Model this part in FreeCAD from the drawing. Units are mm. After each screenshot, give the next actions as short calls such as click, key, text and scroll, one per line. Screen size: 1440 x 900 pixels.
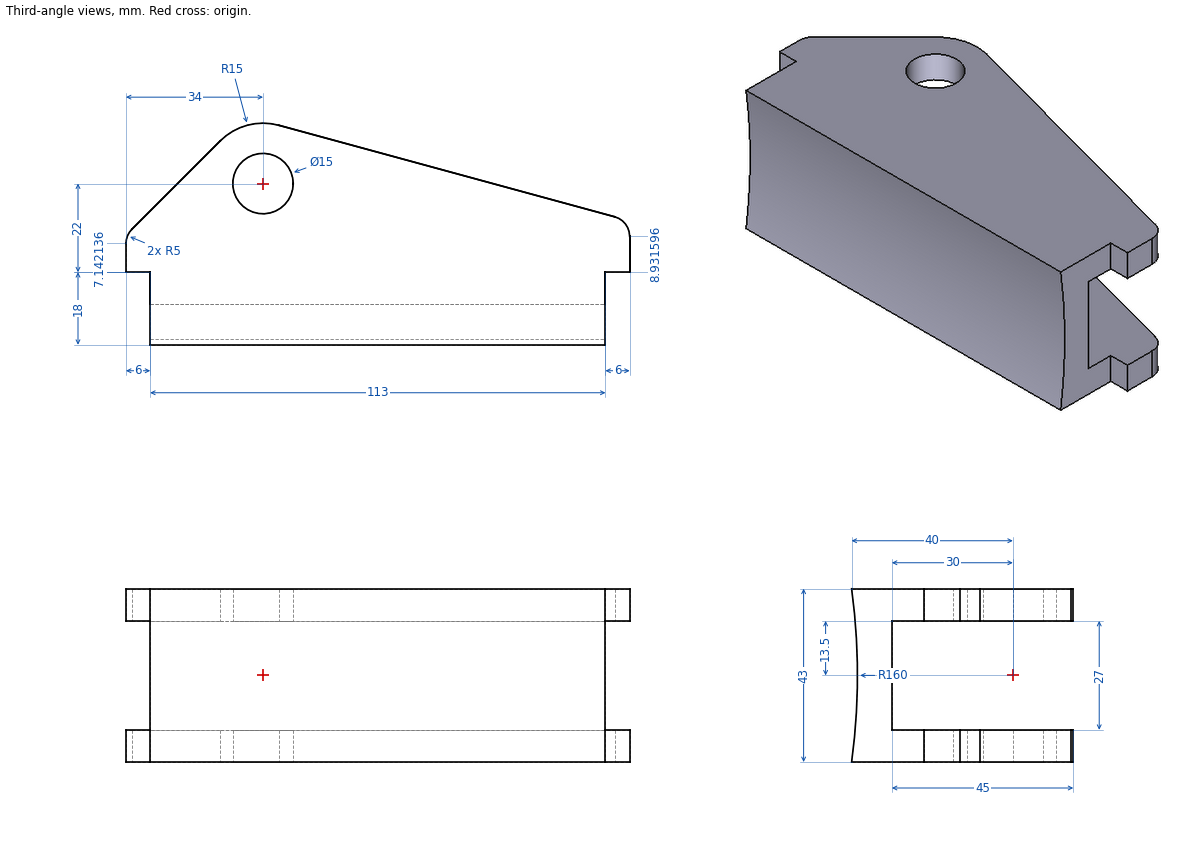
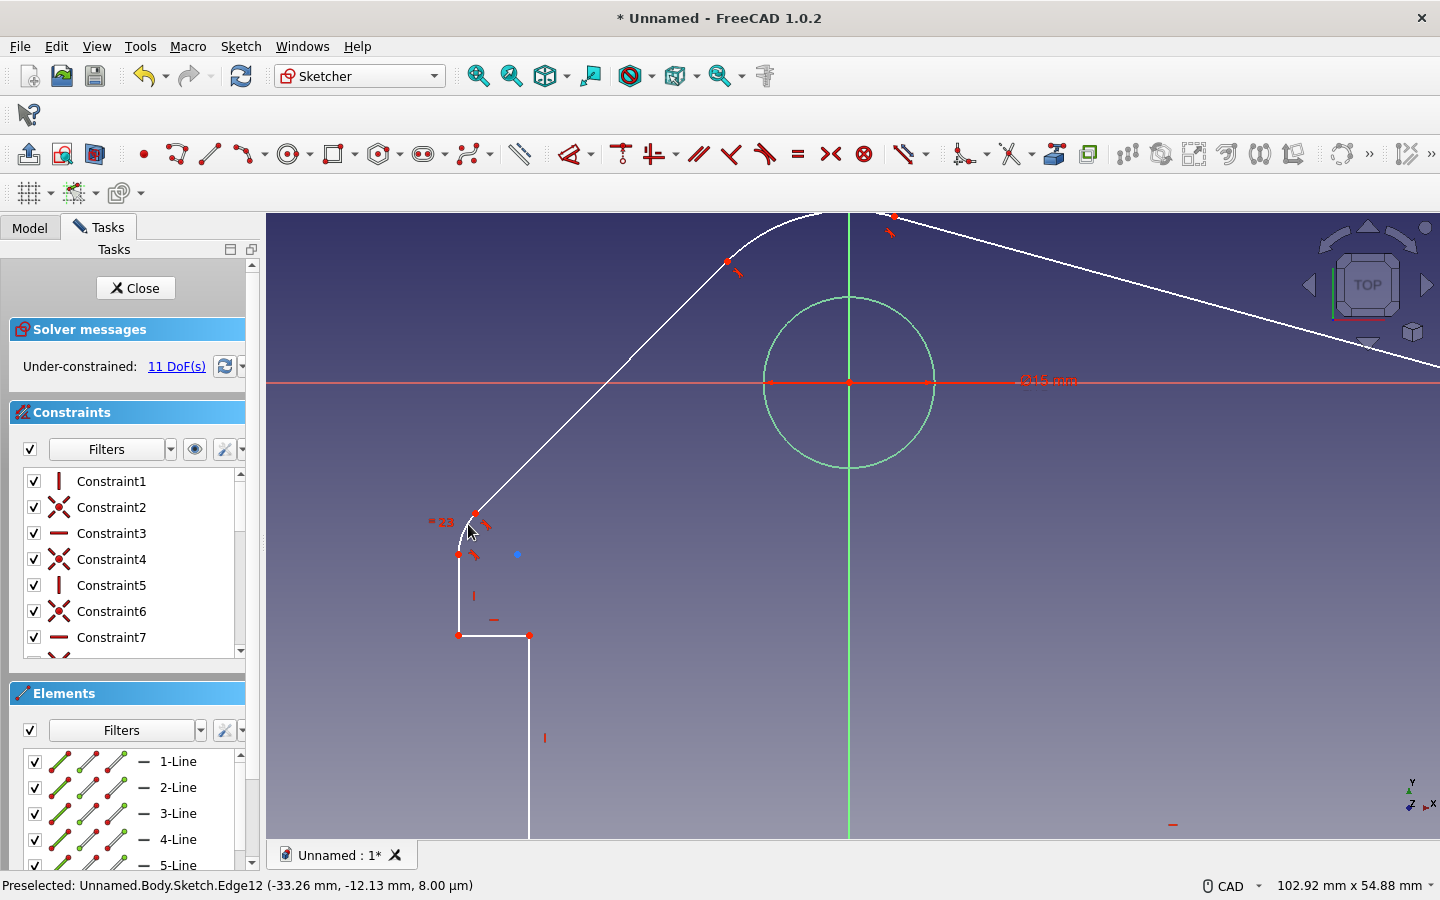
click(568, 154)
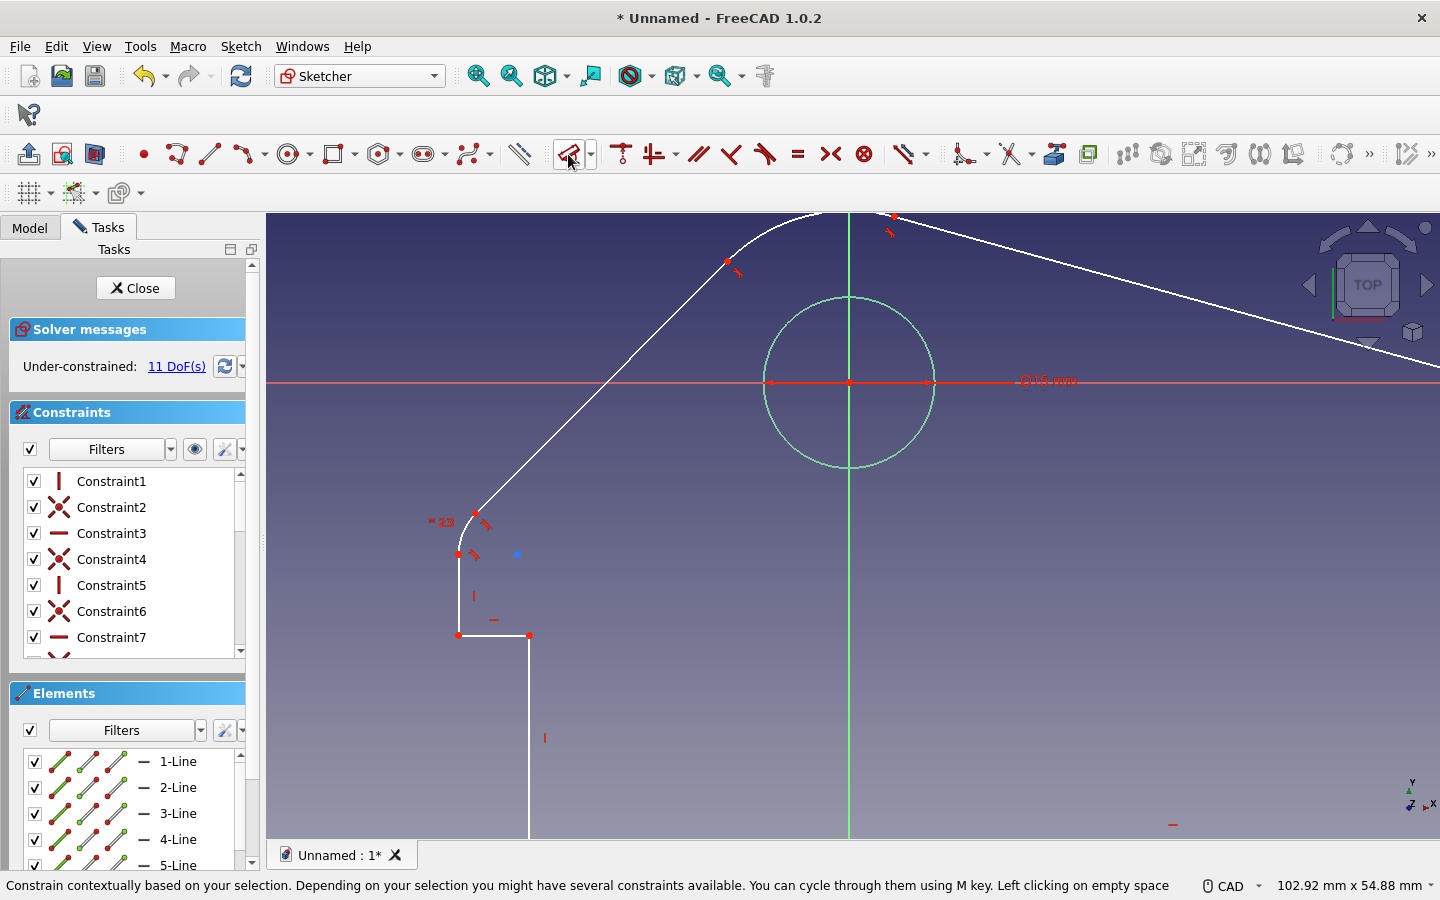
scroll(467, 524, down, 4)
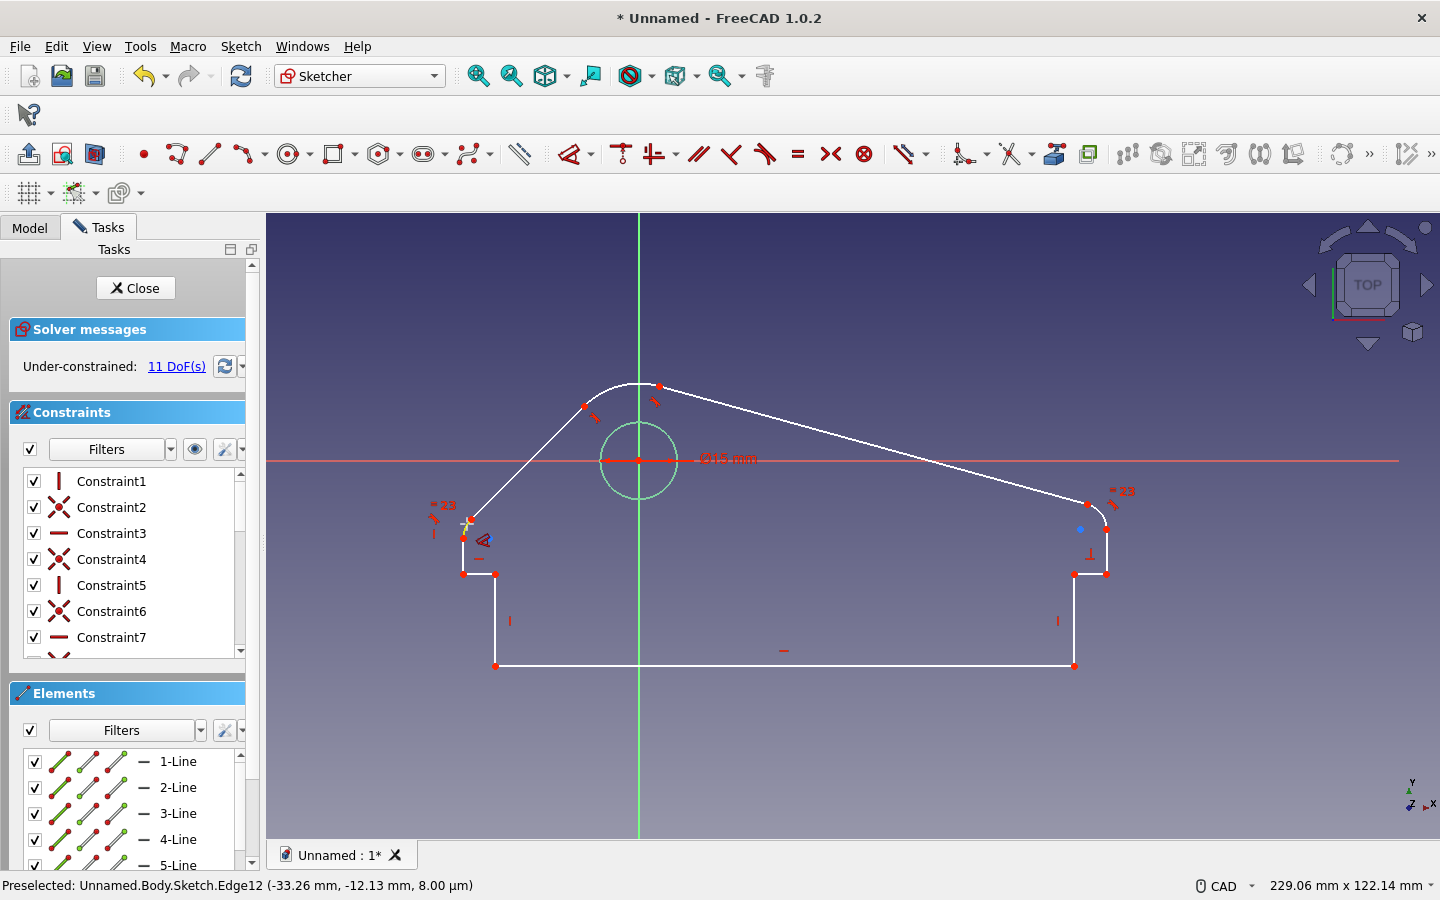
scroll(1105, 520, up, 3)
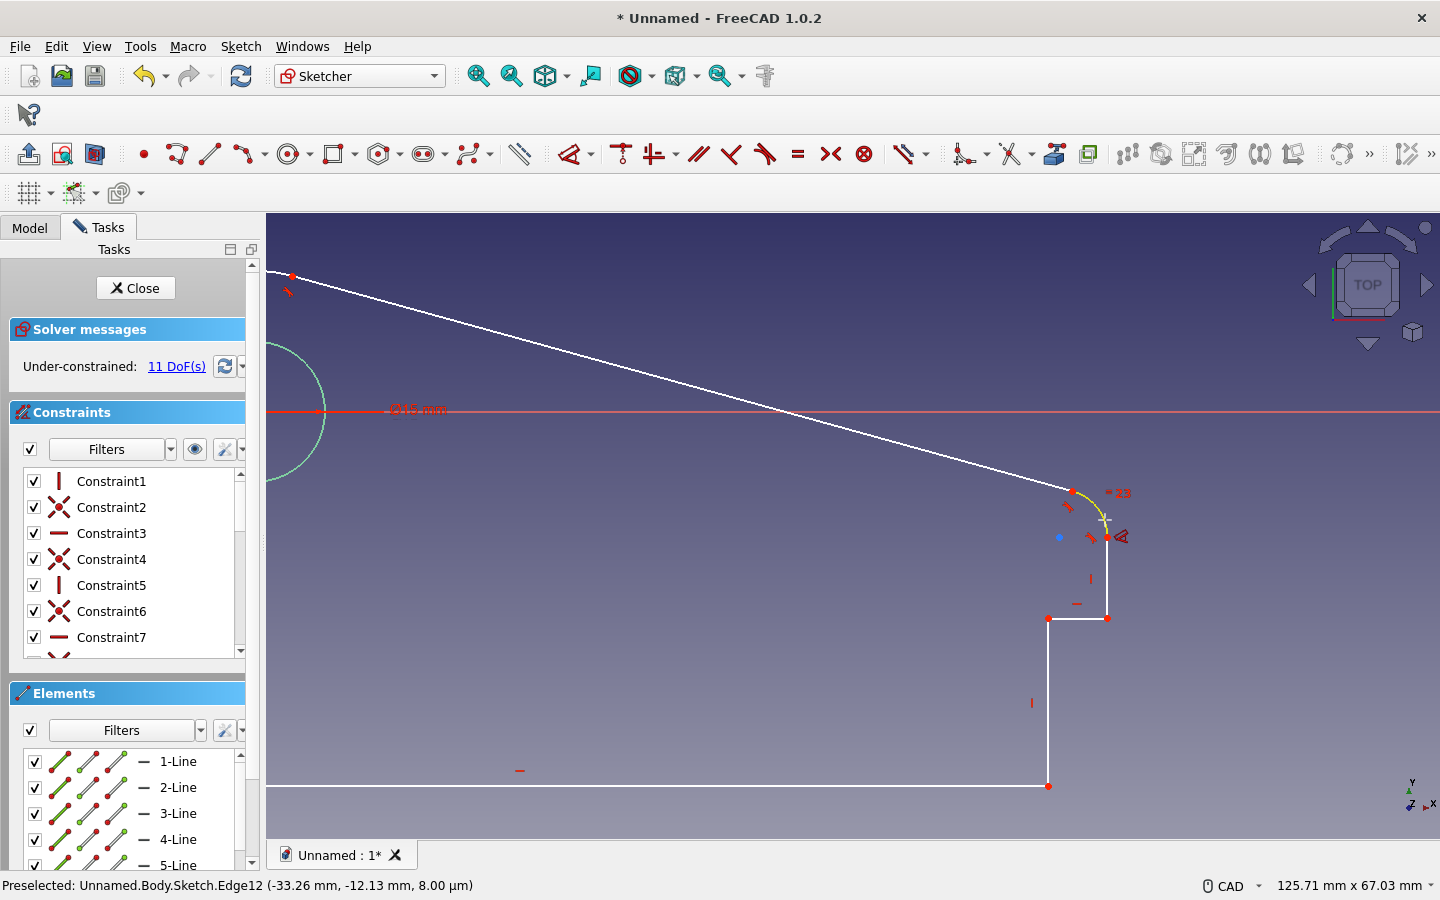
click(1104, 519)
click(1134, 507)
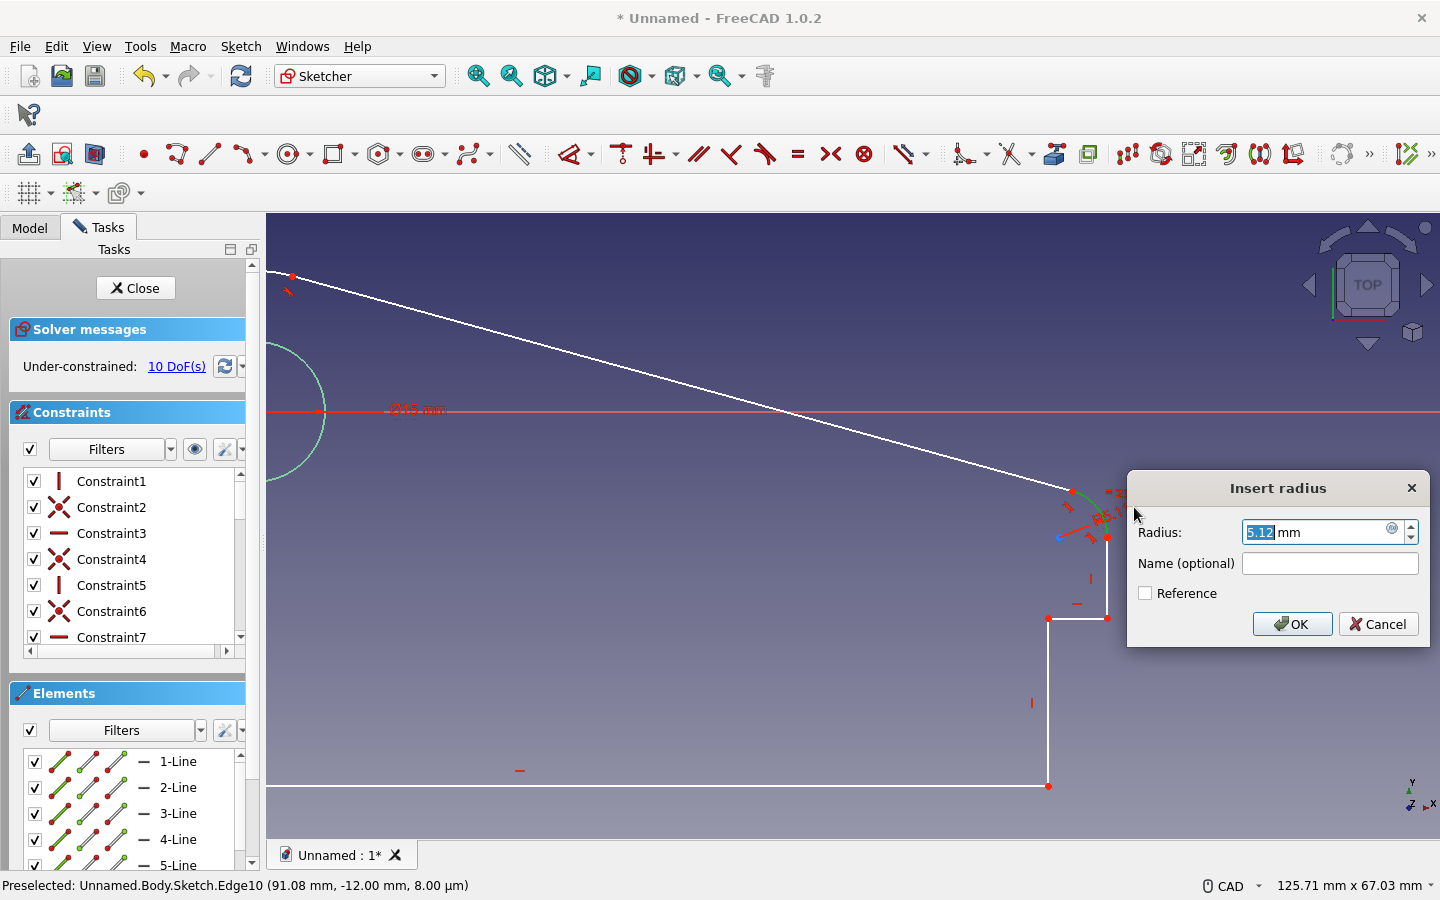
text(5)
key(Return)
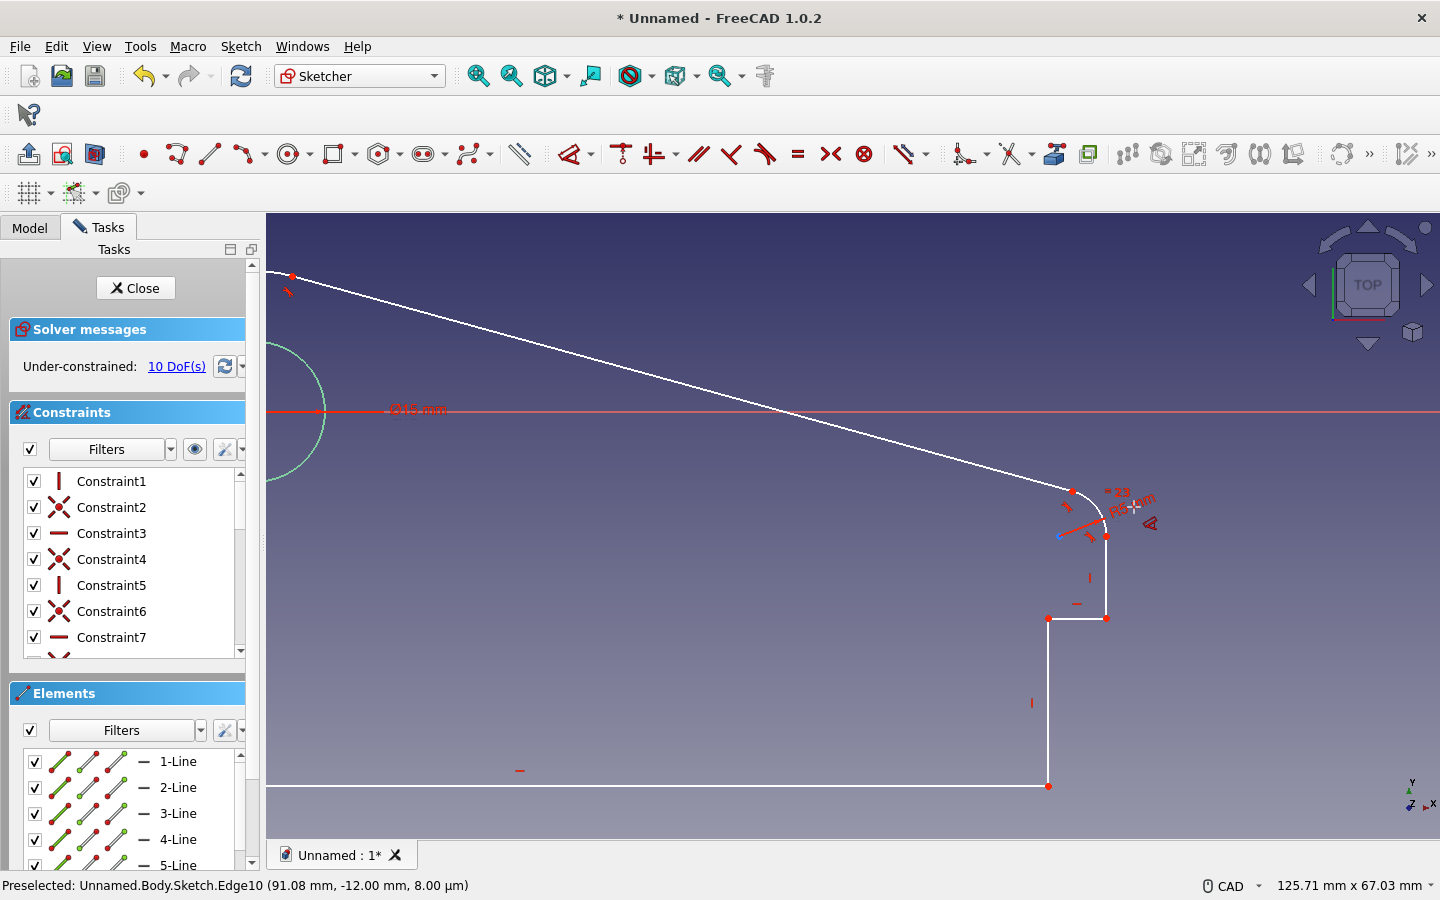
scroll(1105, 520, down, 3)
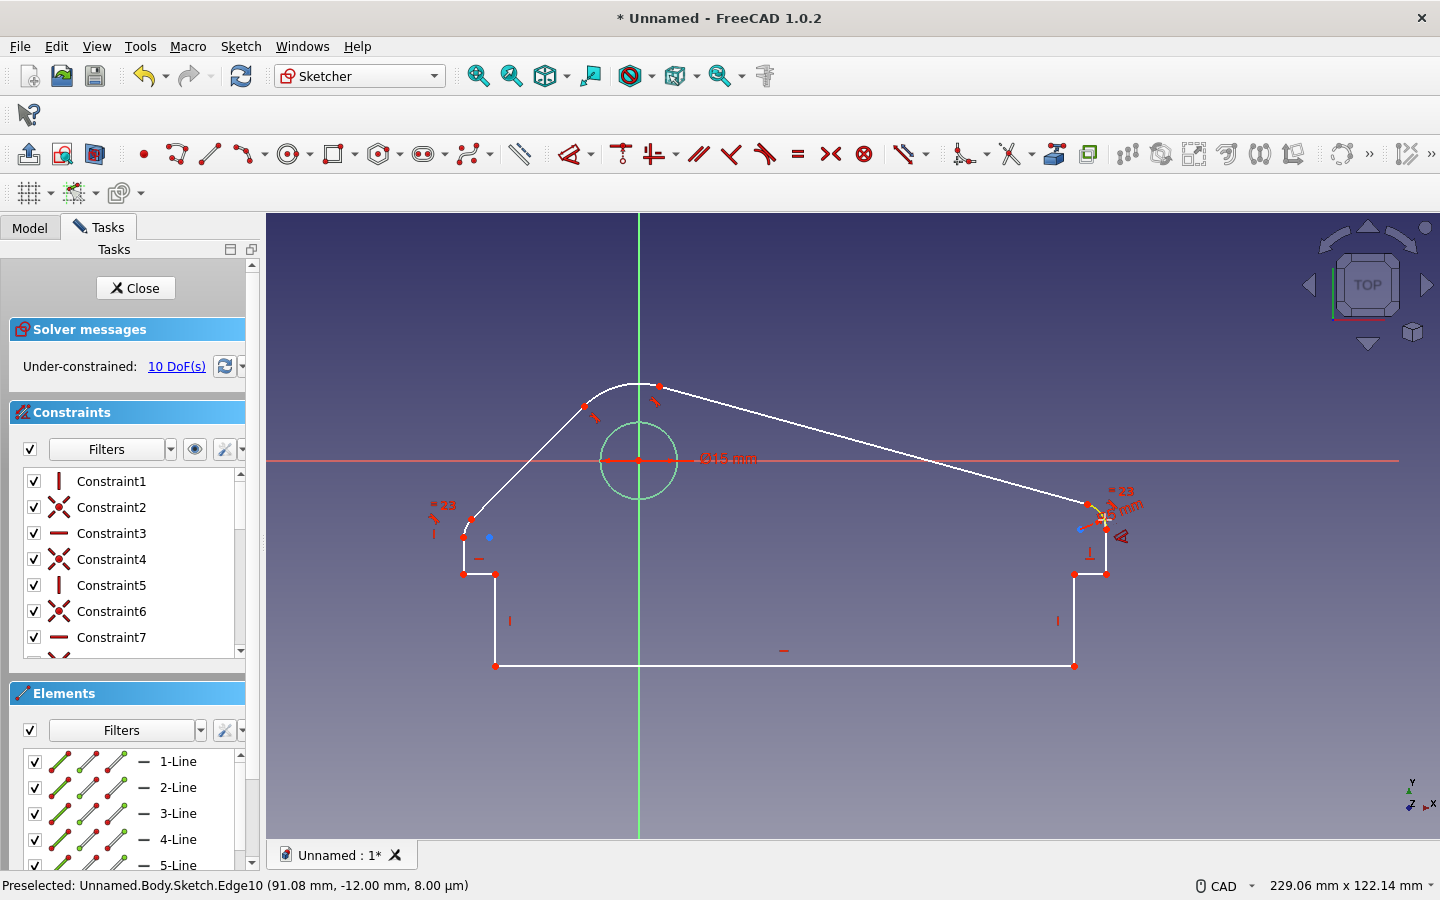
click(604, 392)
click(590, 363)